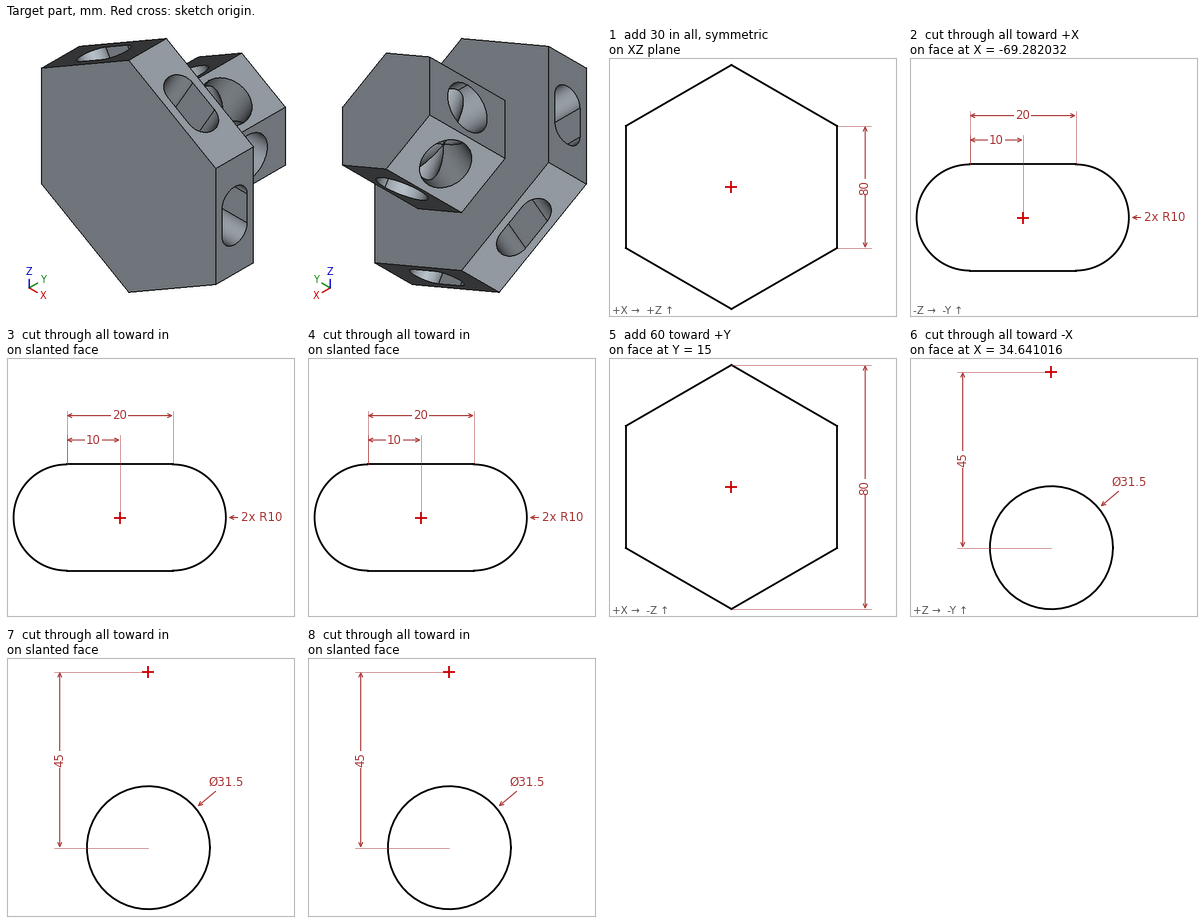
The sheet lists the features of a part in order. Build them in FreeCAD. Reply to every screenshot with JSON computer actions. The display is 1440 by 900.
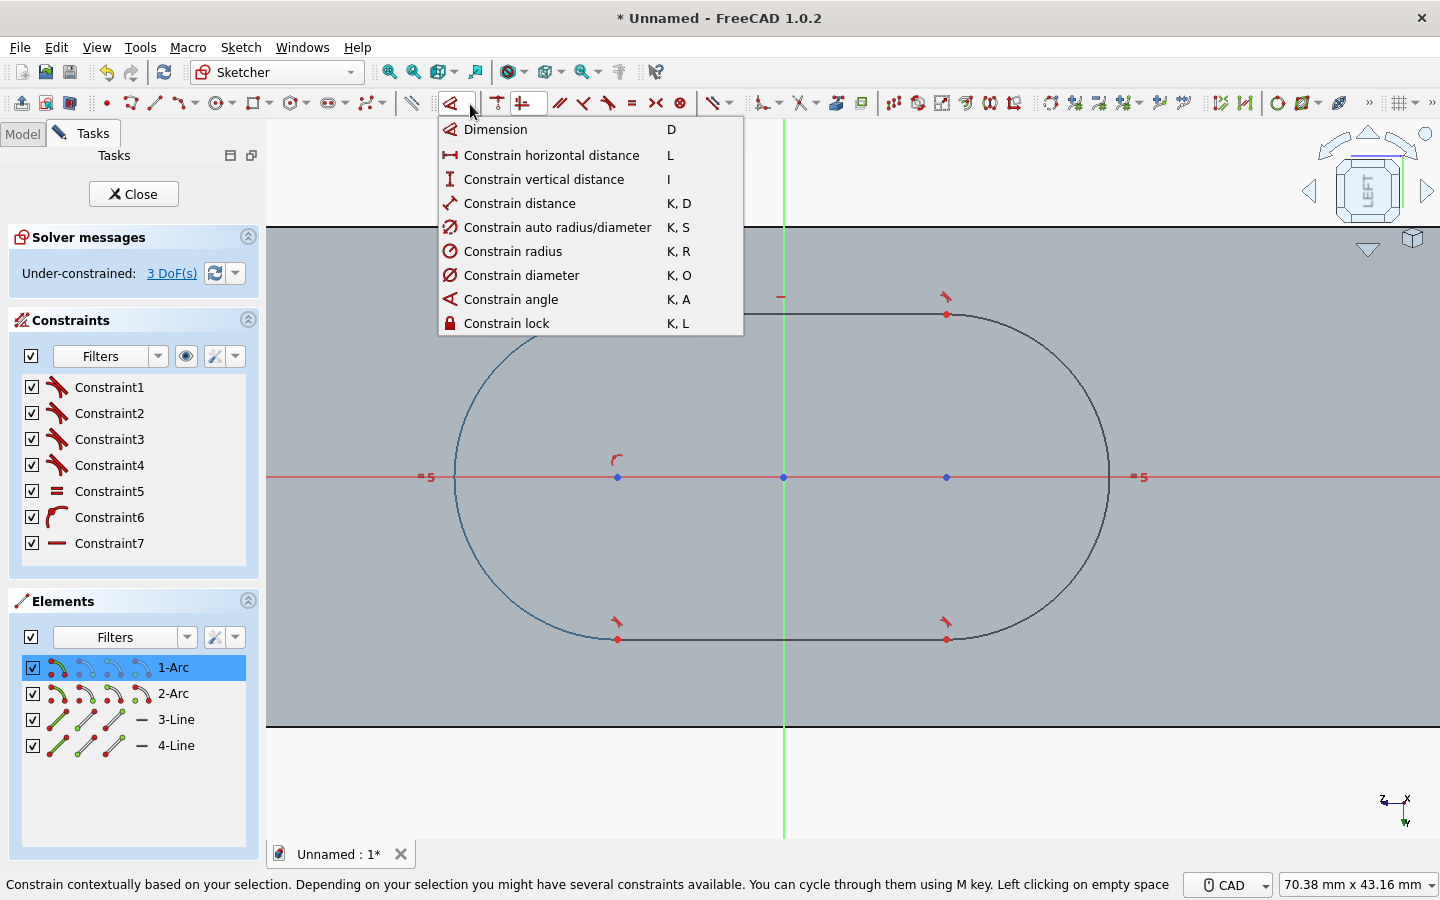
{"action": "left_click", "coordinate": [591, 251]}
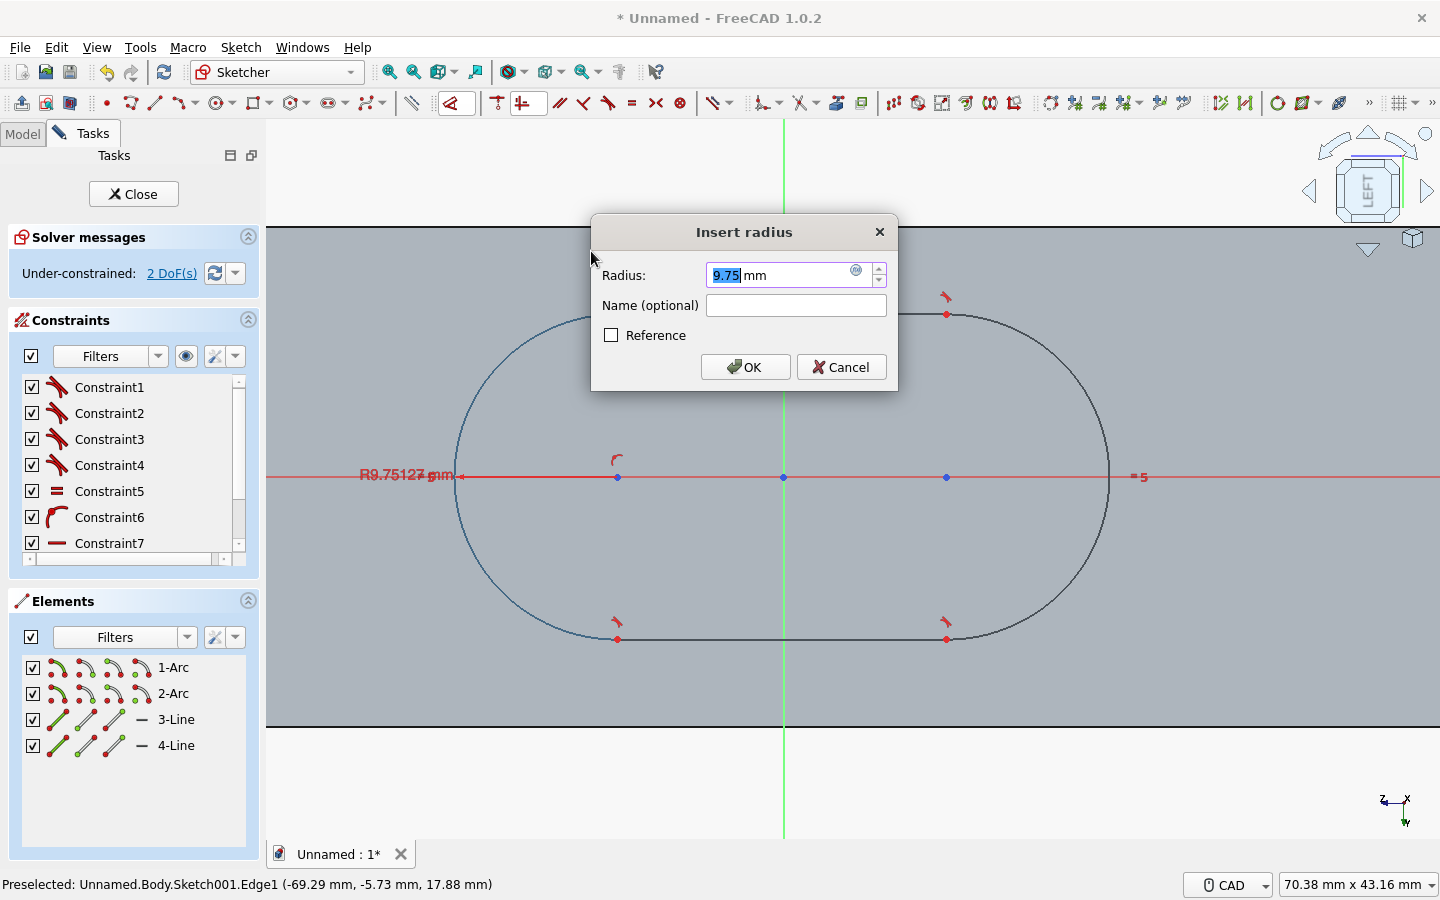
{"action": "type", "text": "10"}
{"action": "key", "text": "Return"}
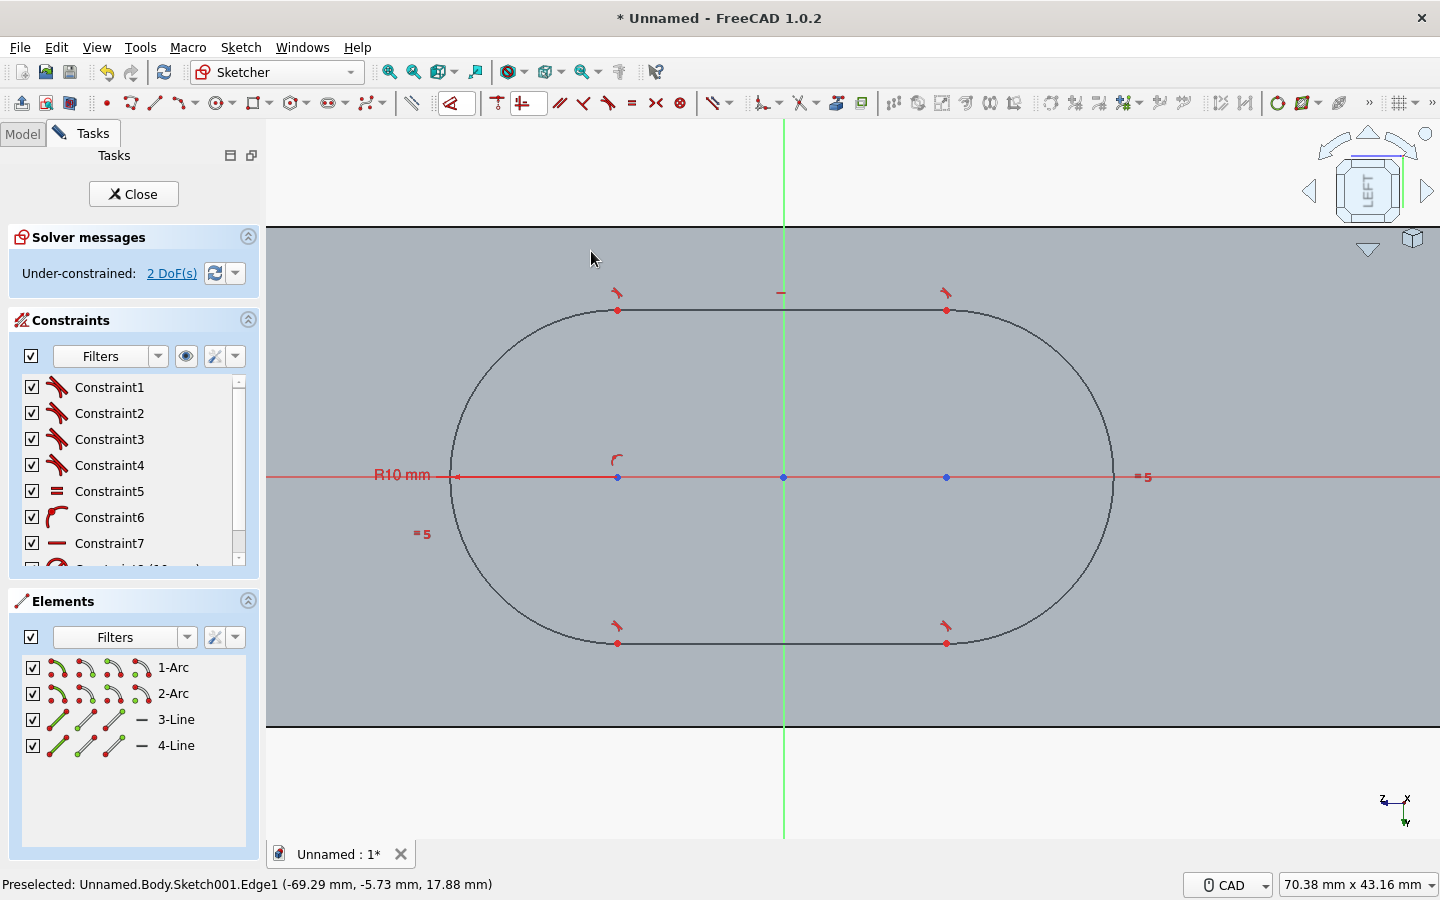
{"action": "left_click", "coordinate": [716, 310]}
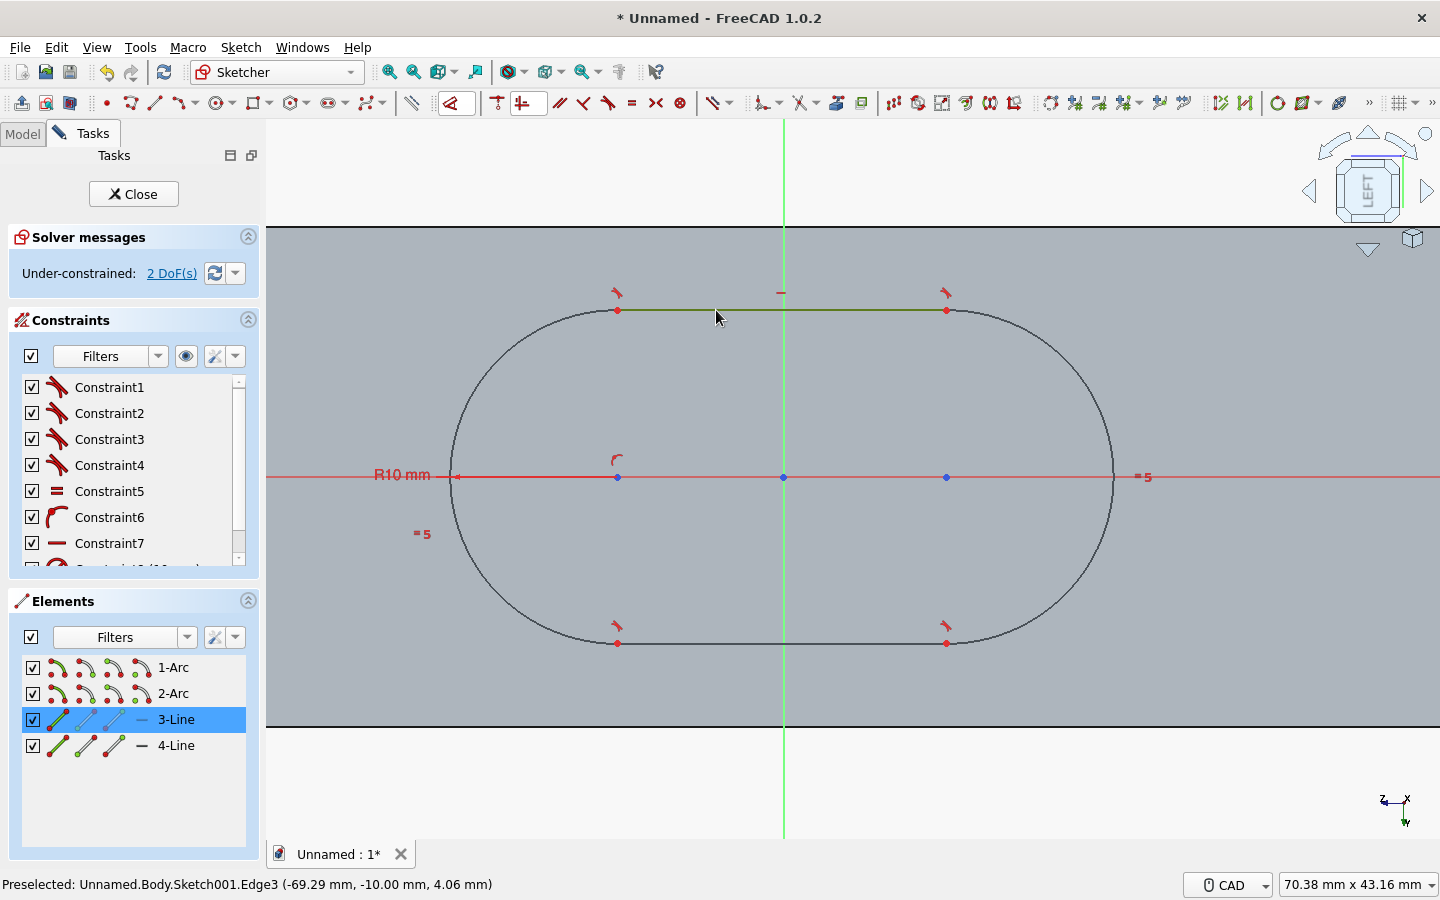
{"action": "left_click", "coordinate": [470, 104]}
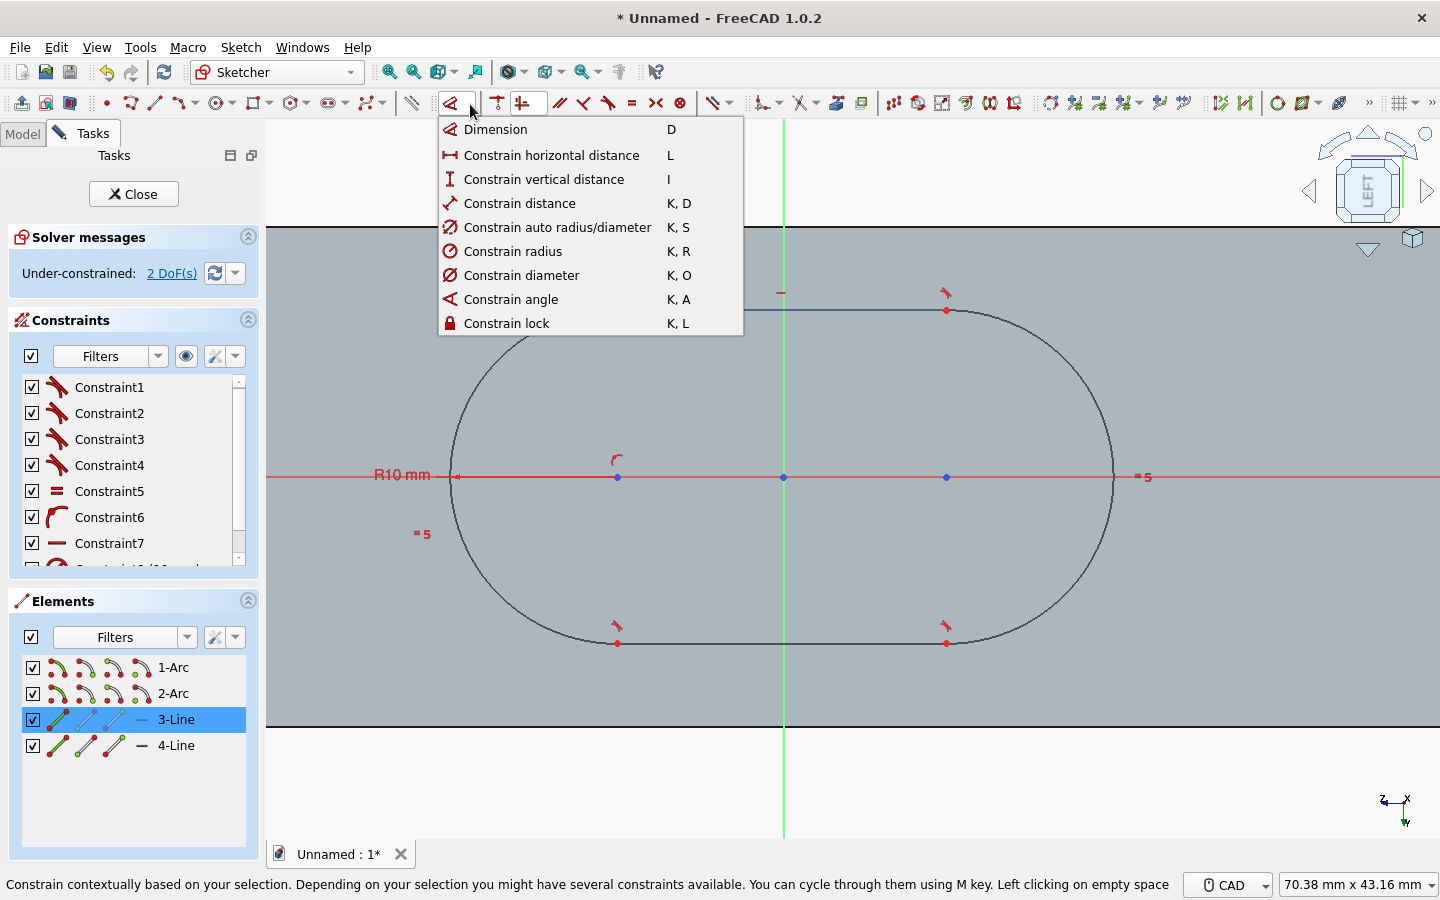
{"action": "left_click", "coordinate": [591, 155]}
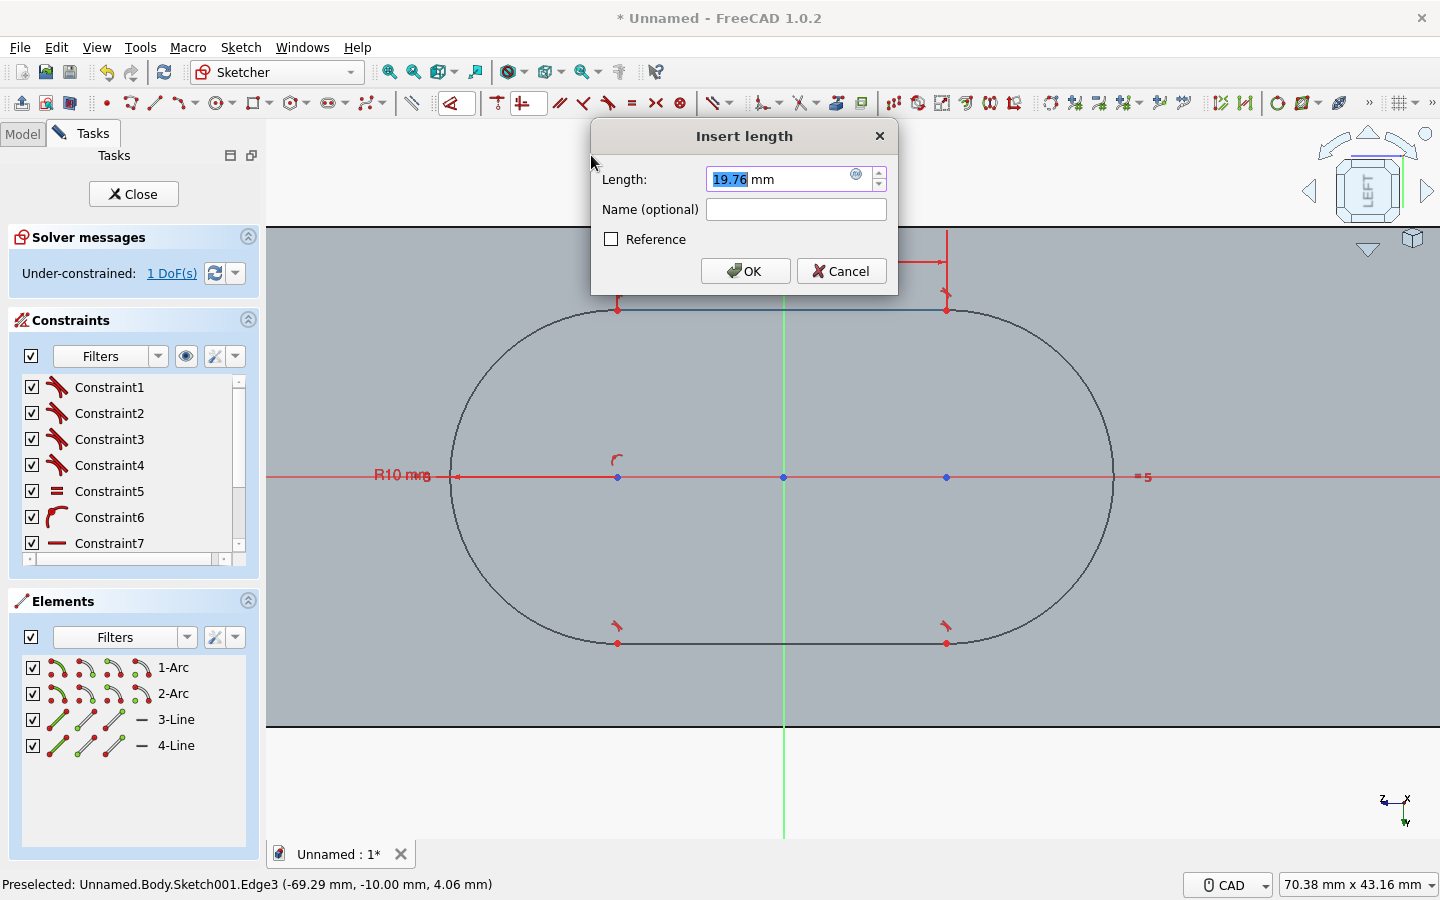
{"action": "type", "text": "20"}
{"action": "key", "text": "Return"}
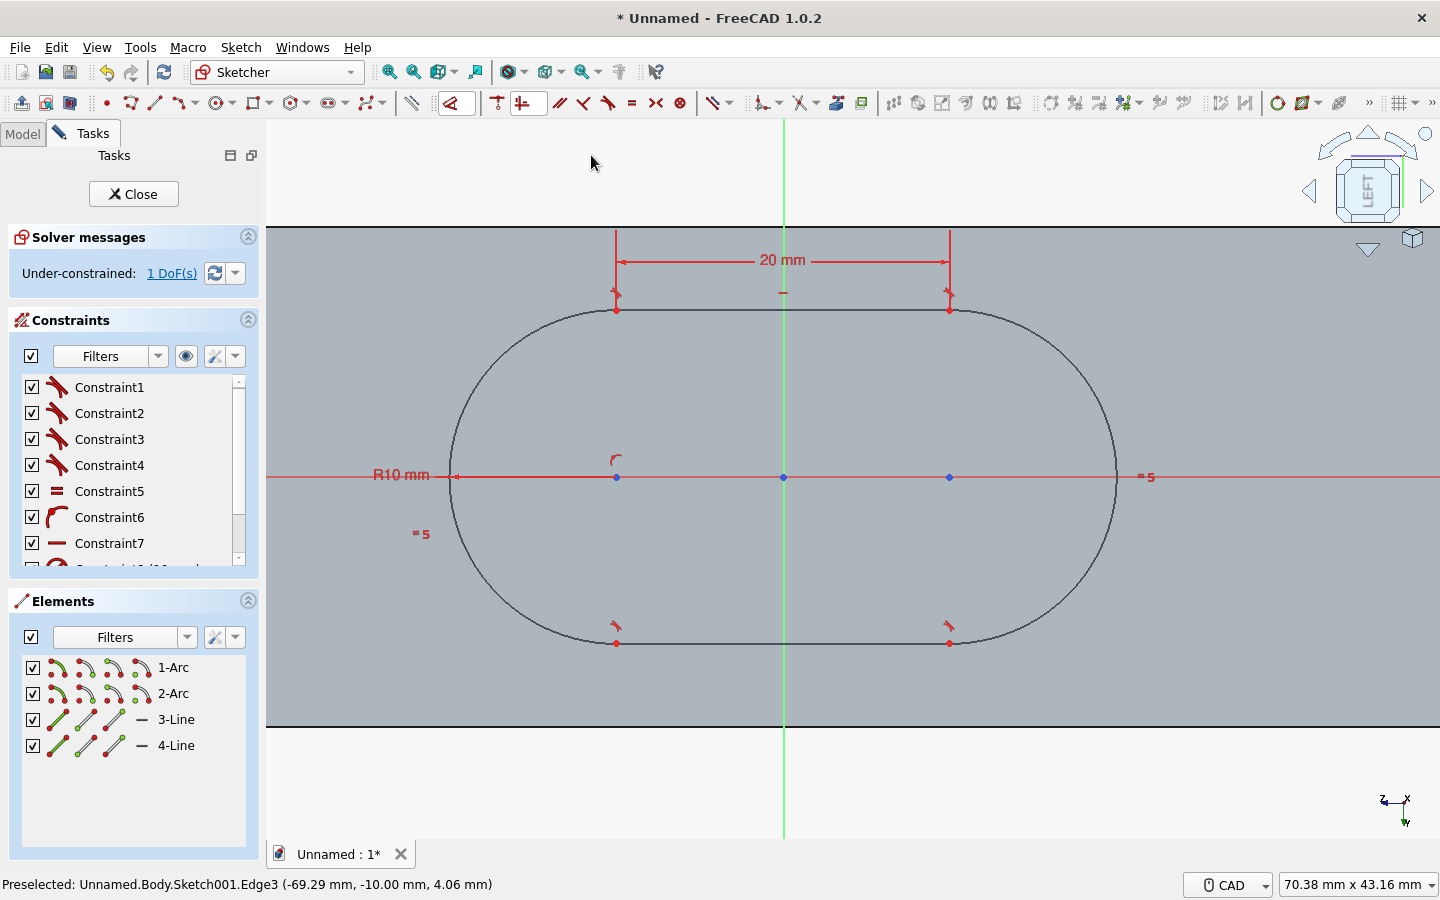
{"action": "left_click", "coordinate": [616, 310]}